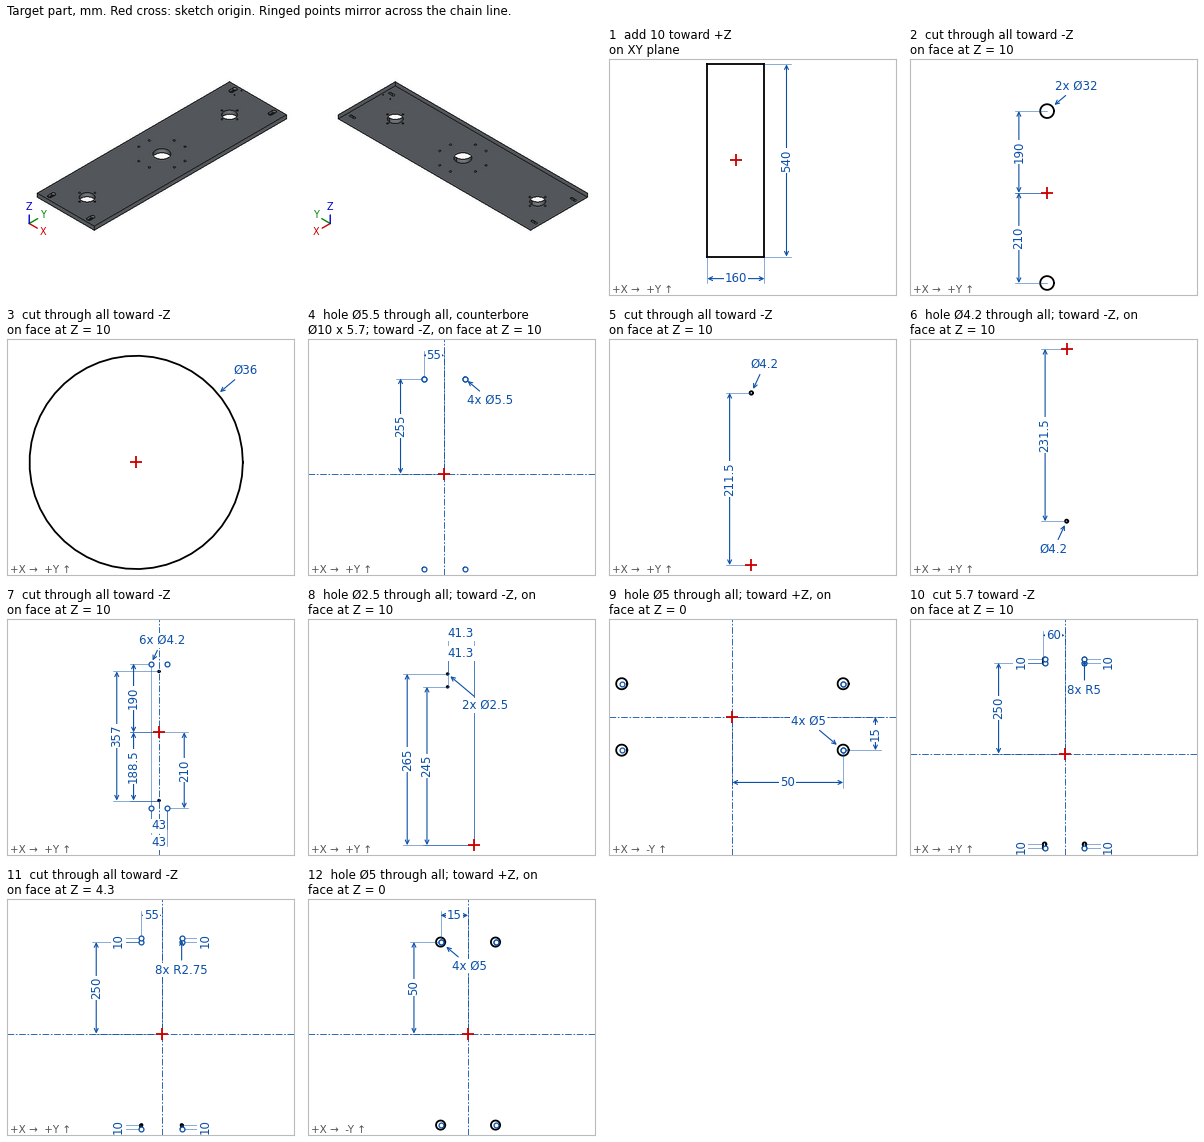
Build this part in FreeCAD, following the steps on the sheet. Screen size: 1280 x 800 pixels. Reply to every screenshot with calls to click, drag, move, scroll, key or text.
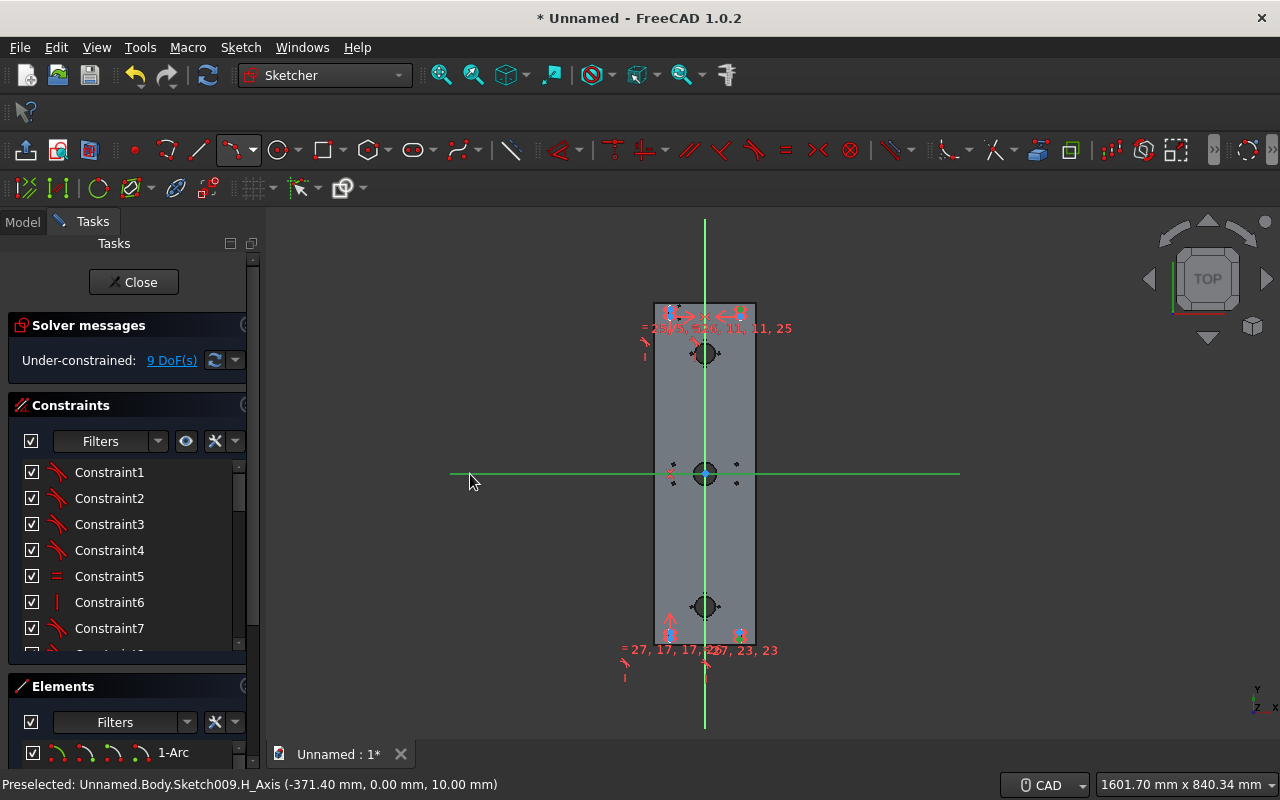
key(s)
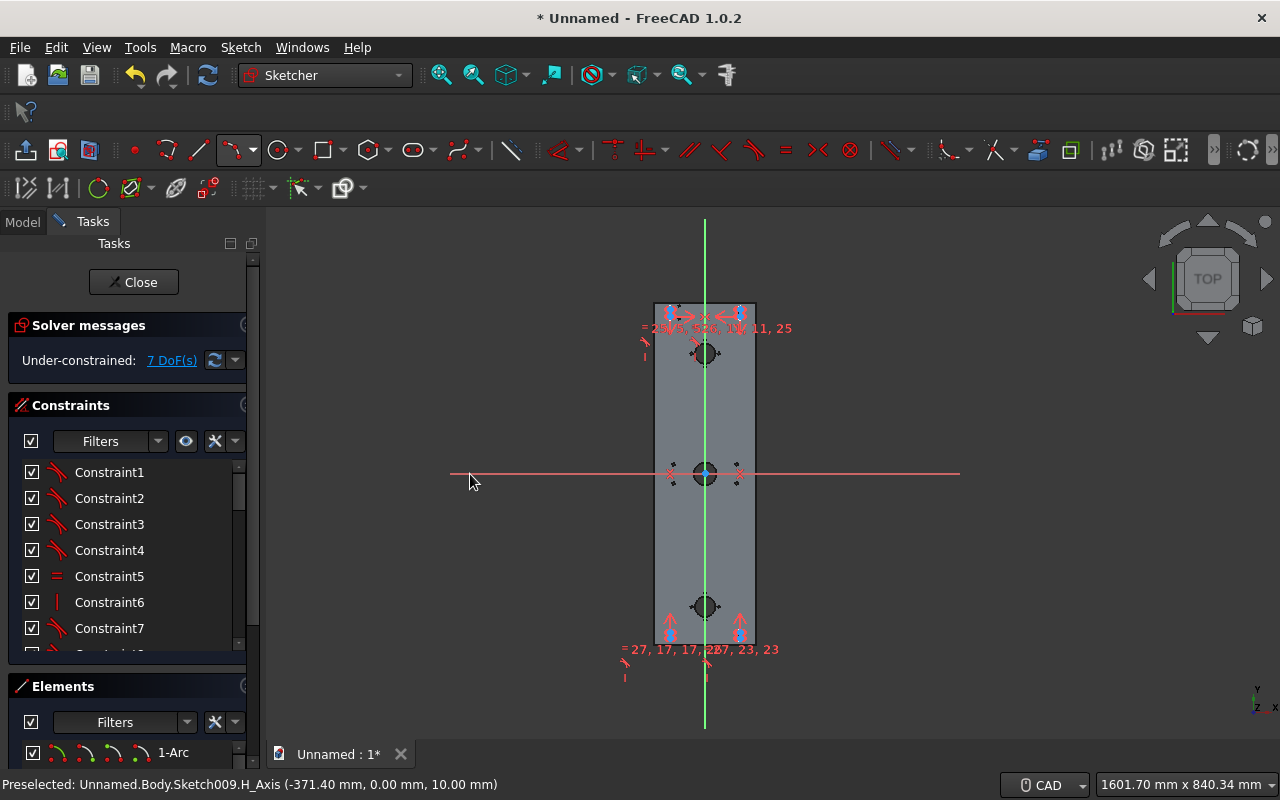
click(558, 150)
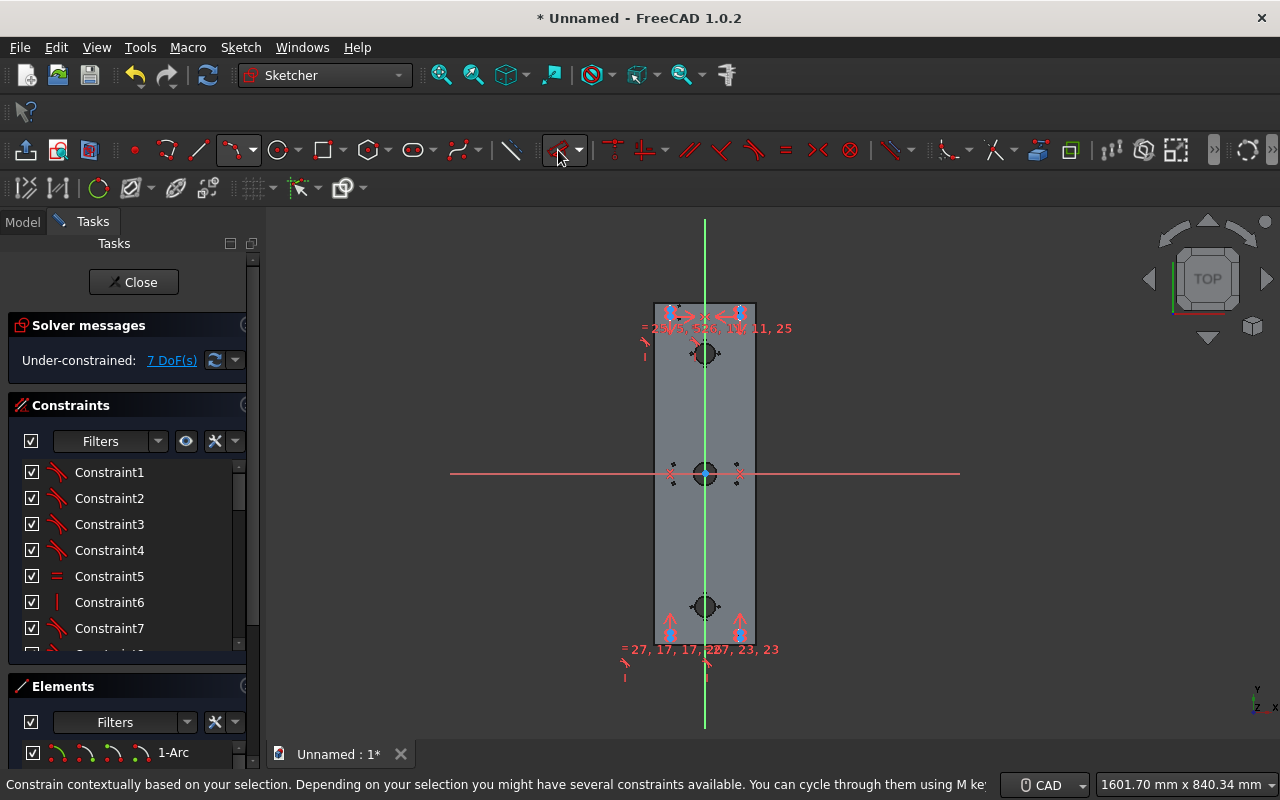
scroll(670, 320, up, 13)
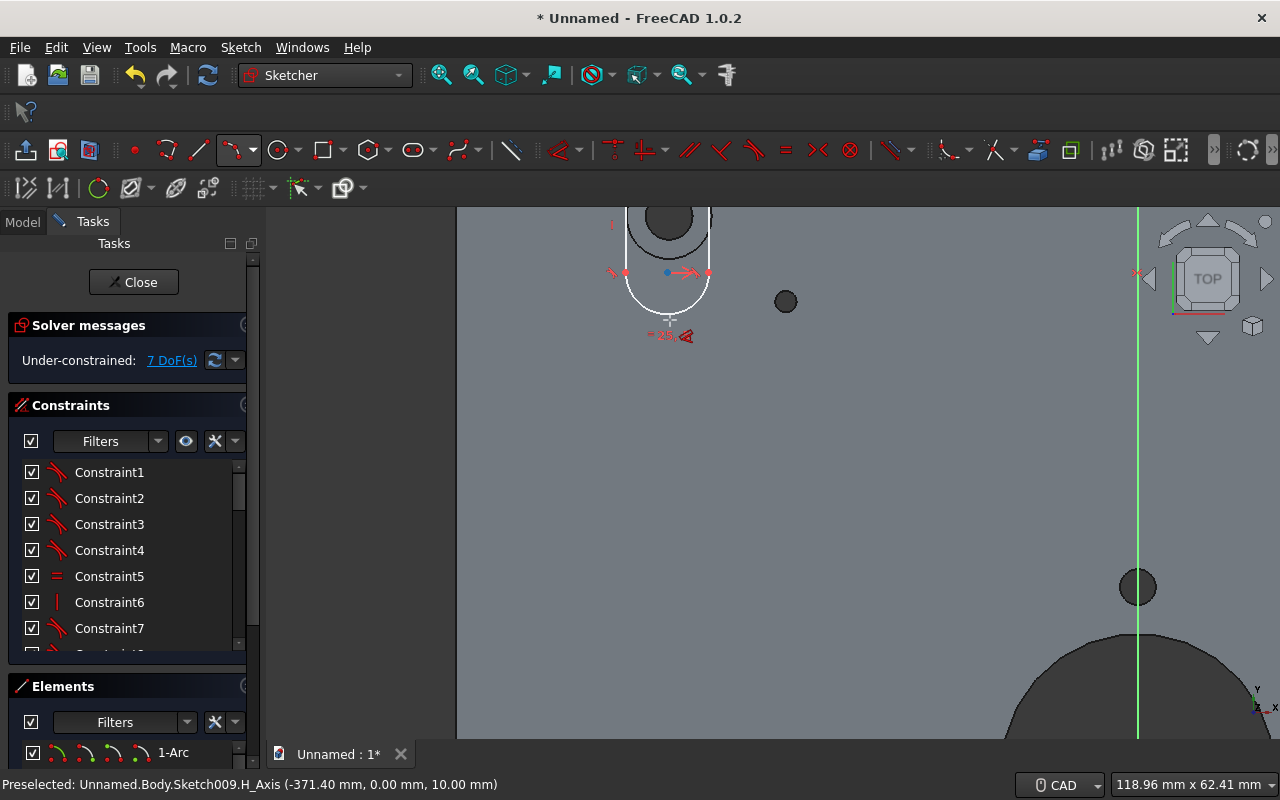
click(667, 314)
click(667, 346)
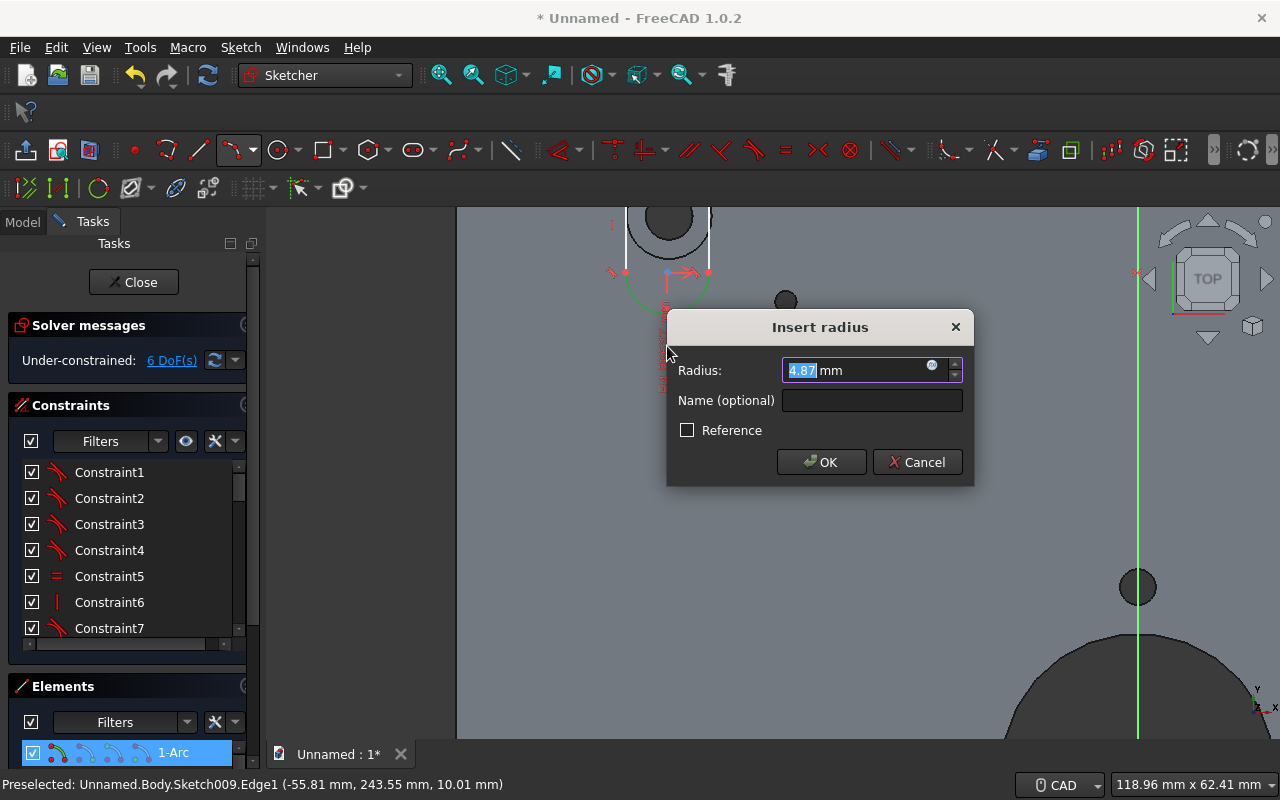
text(5)
key(Return)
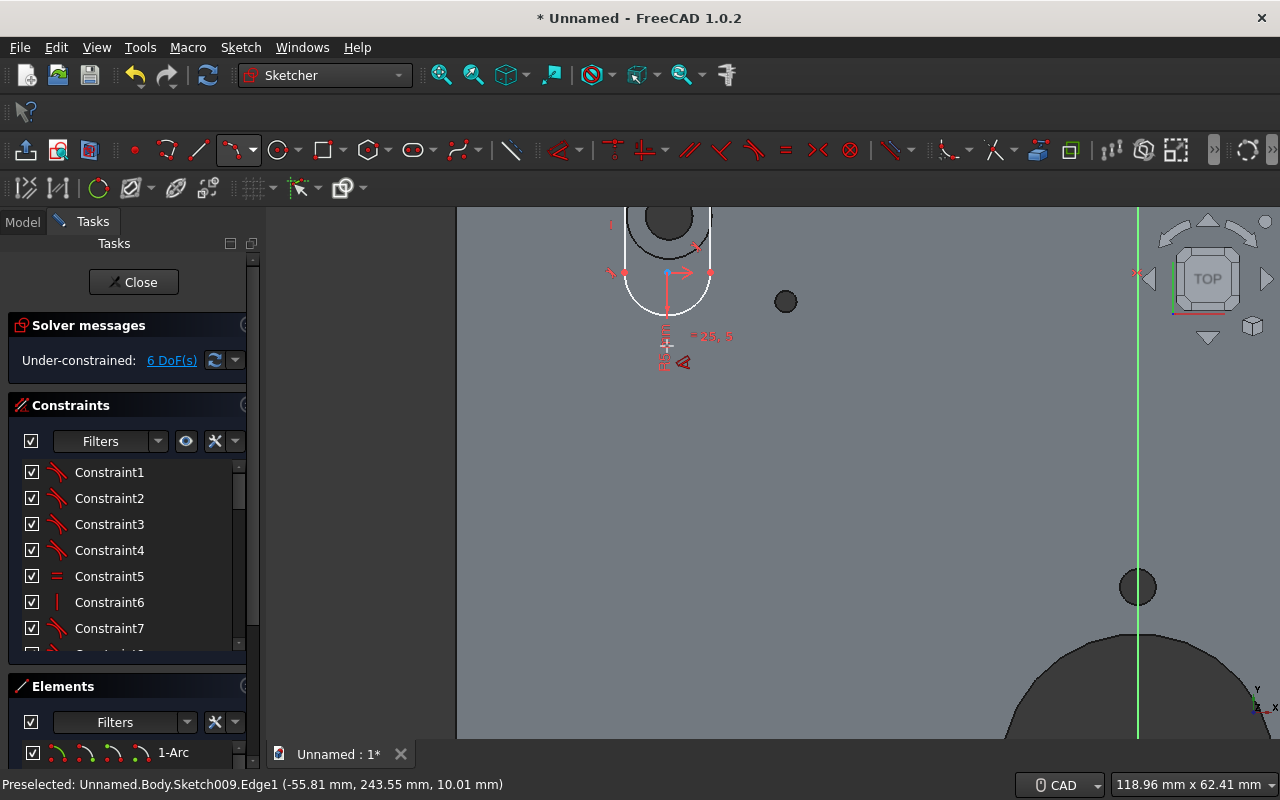
click(625, 244)
click(591, 254)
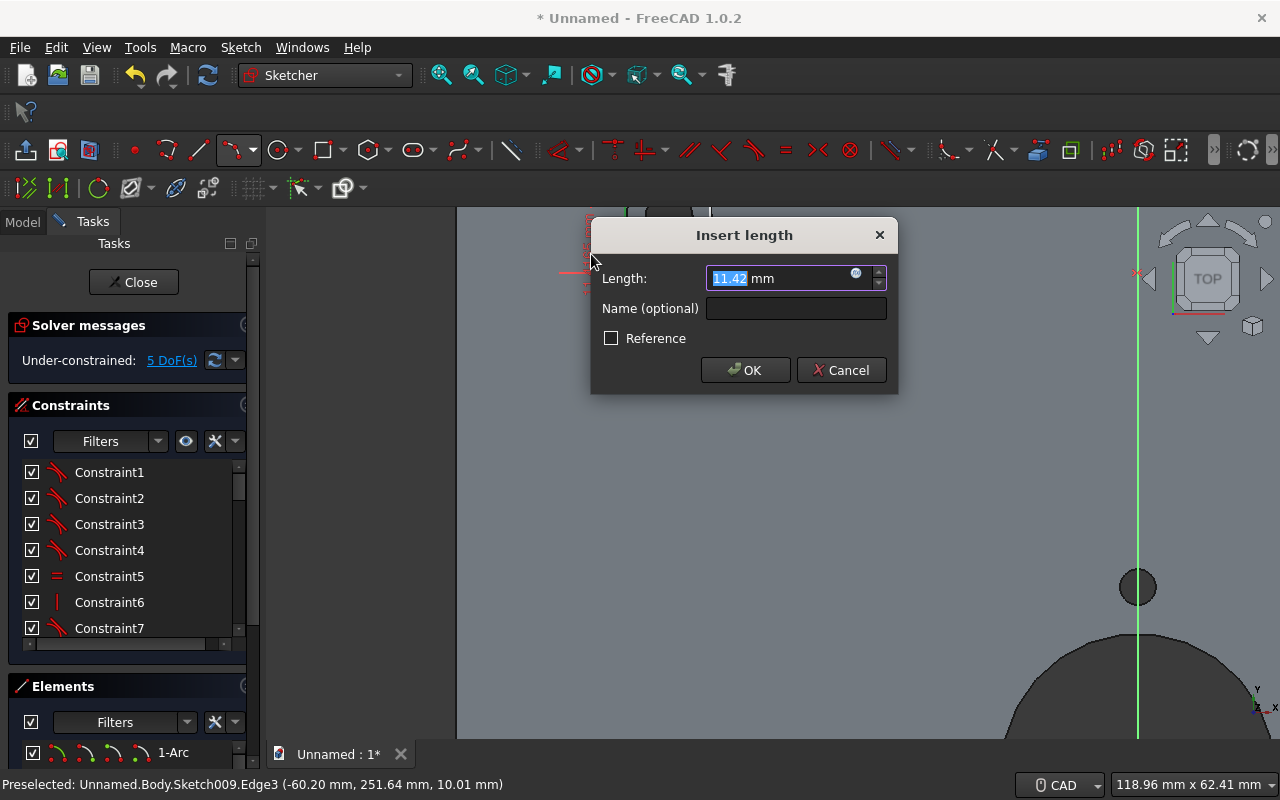
text(10)
key(Return)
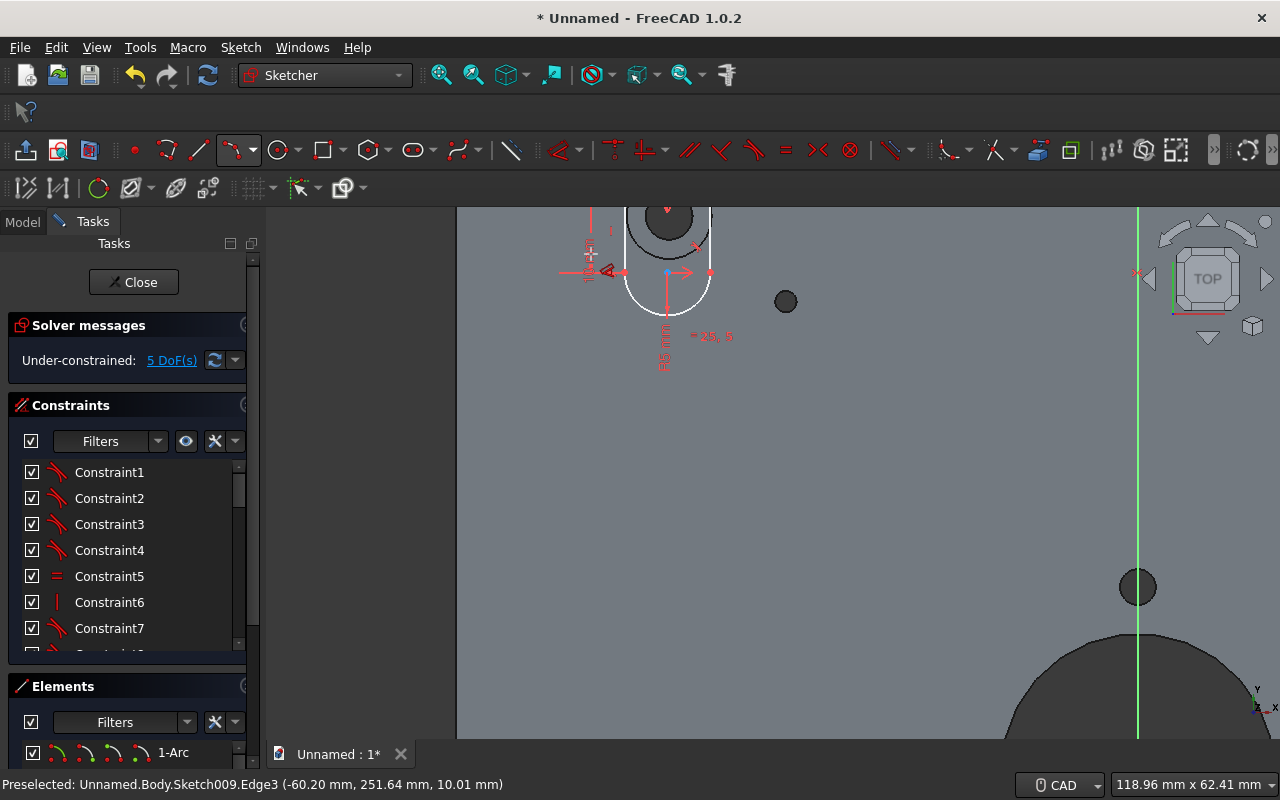
scroll(670, 319, down, 13)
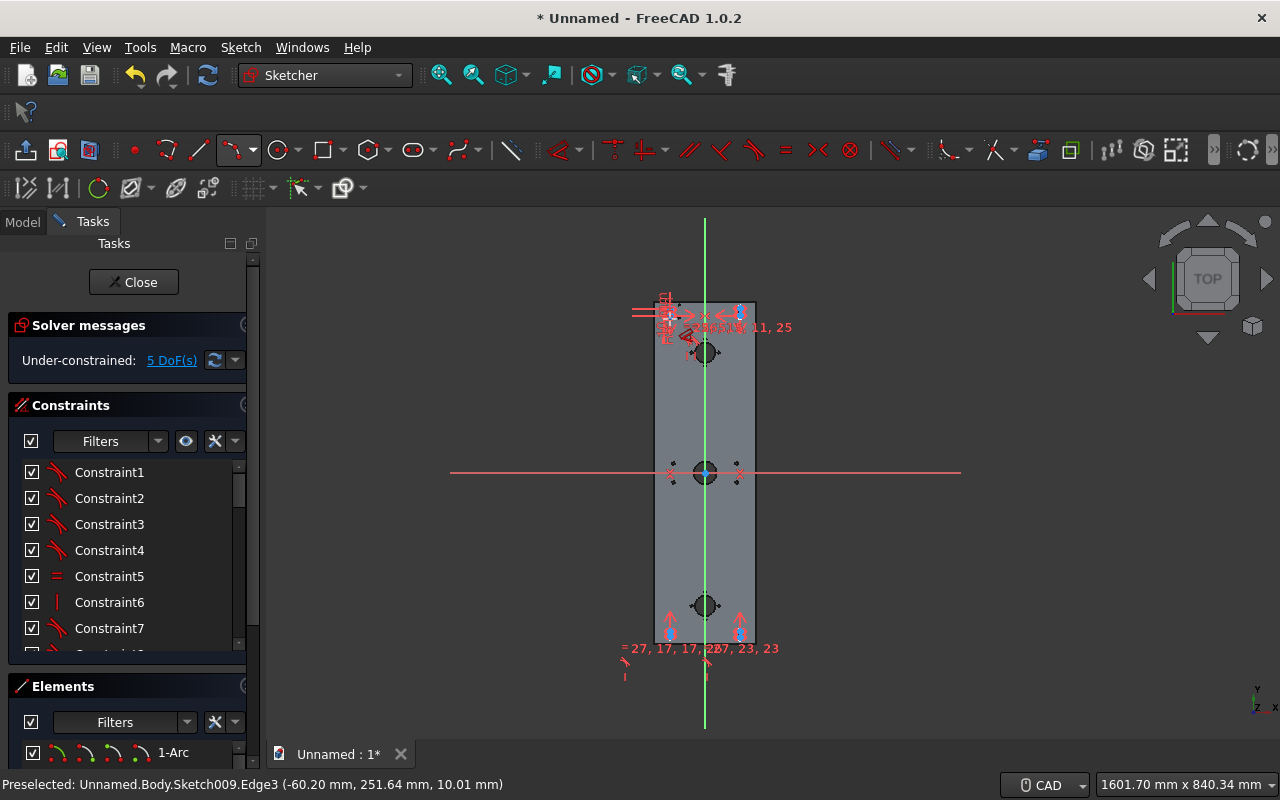
scroll(737, 314, up, 10)